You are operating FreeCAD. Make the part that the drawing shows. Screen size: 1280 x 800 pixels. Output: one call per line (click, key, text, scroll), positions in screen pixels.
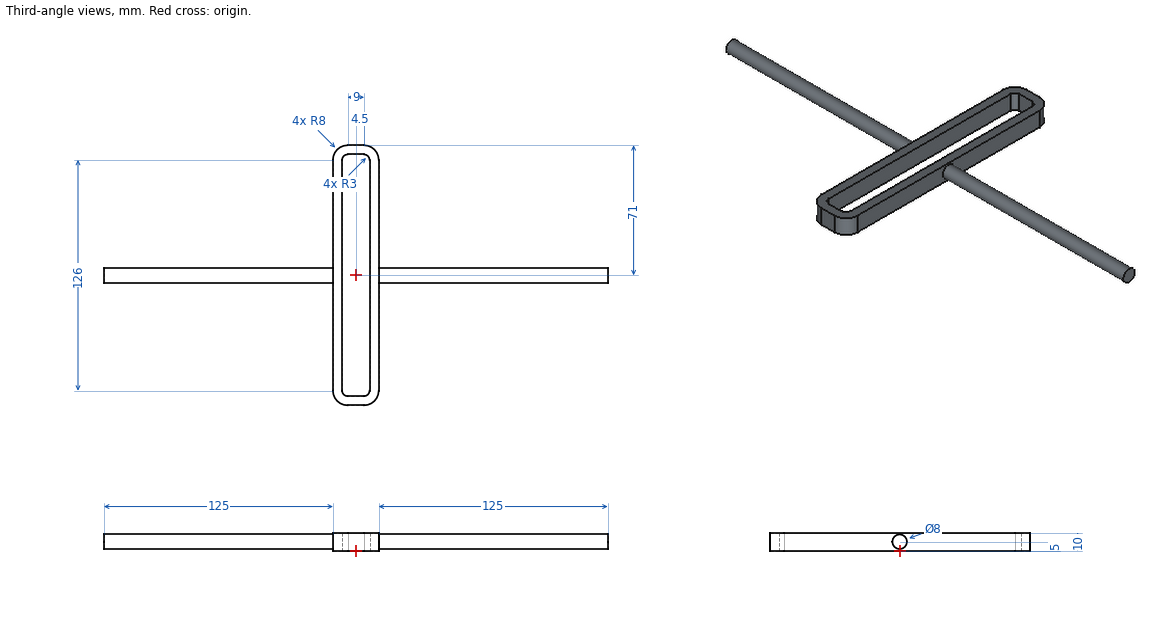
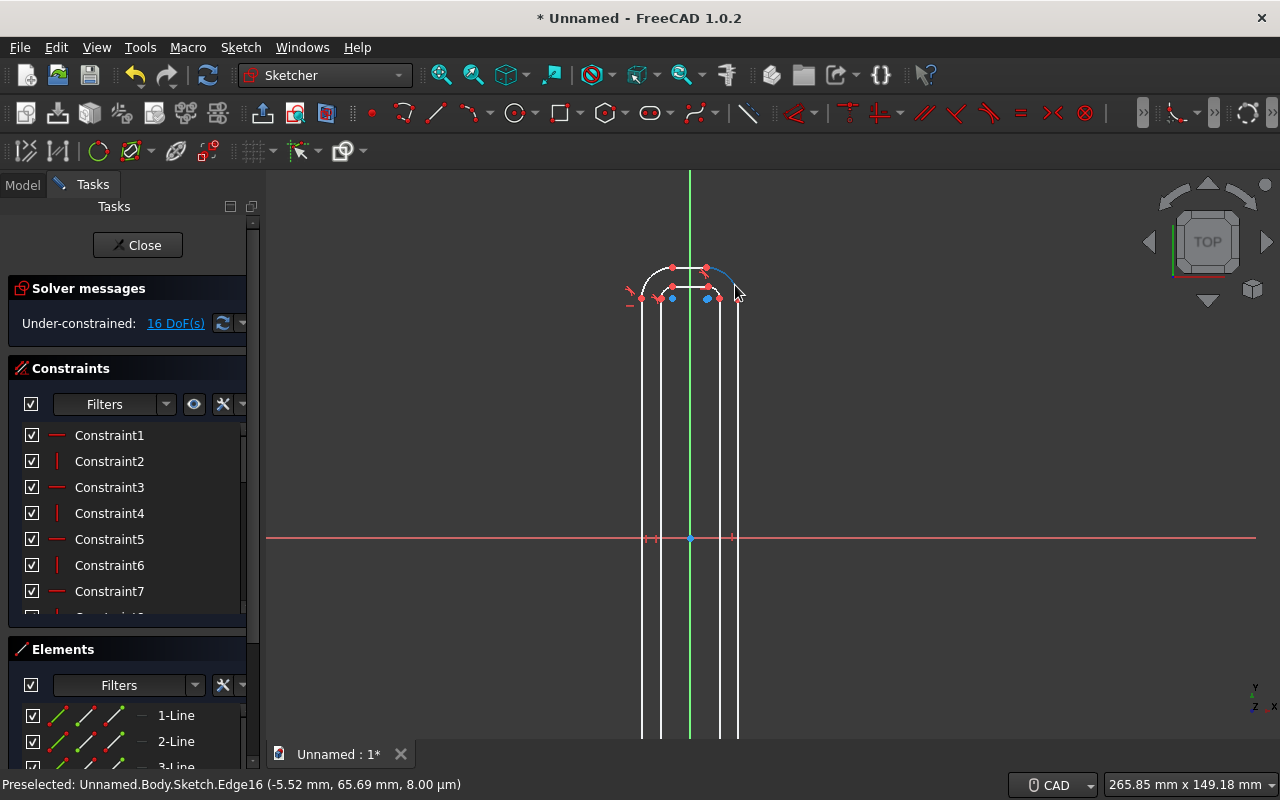
click(734, 285)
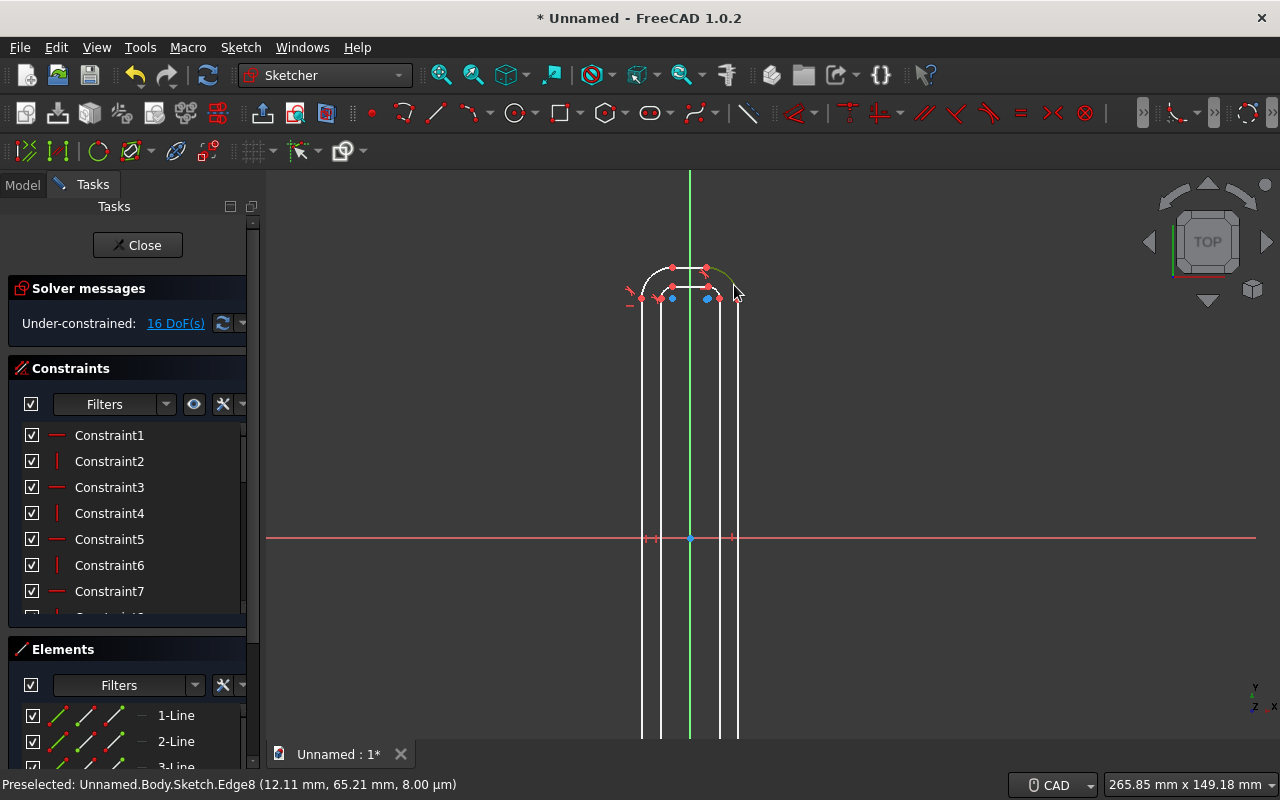
scroll(716, 290, up, 3)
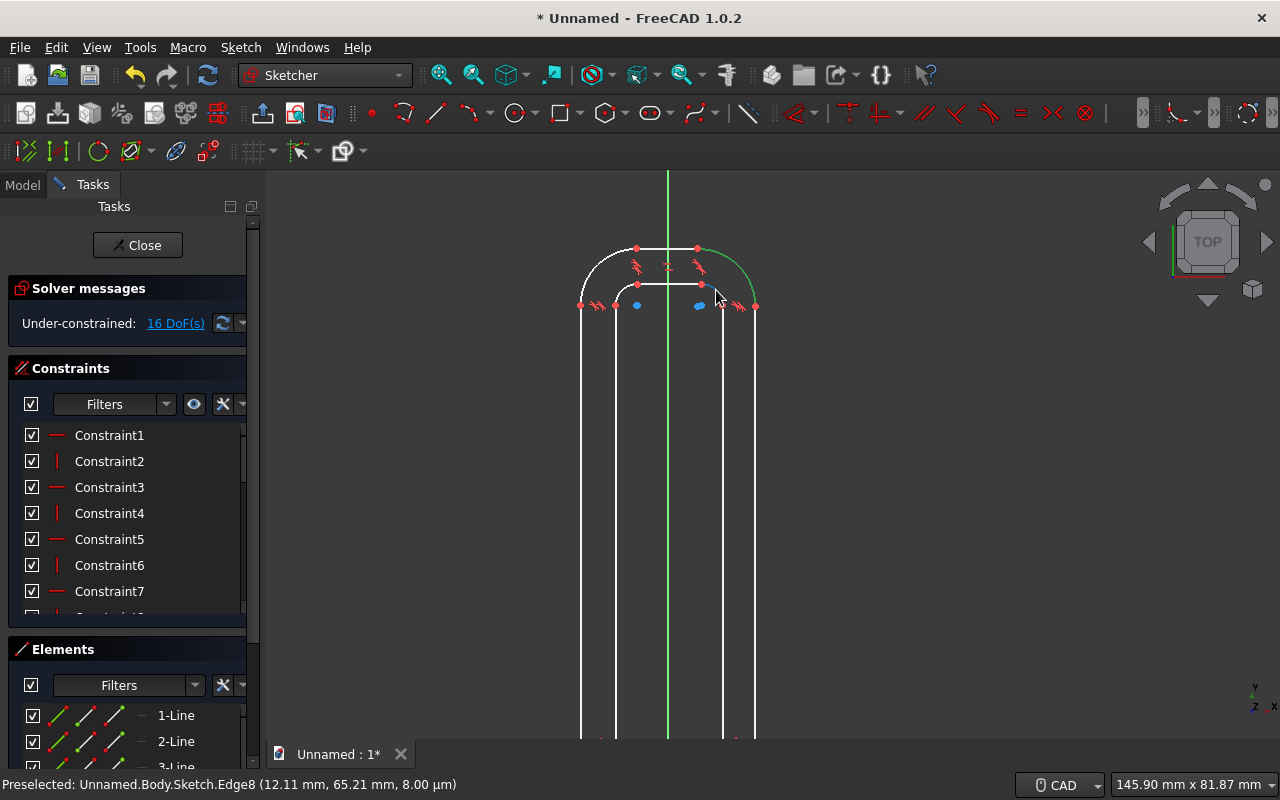
click(716, 290)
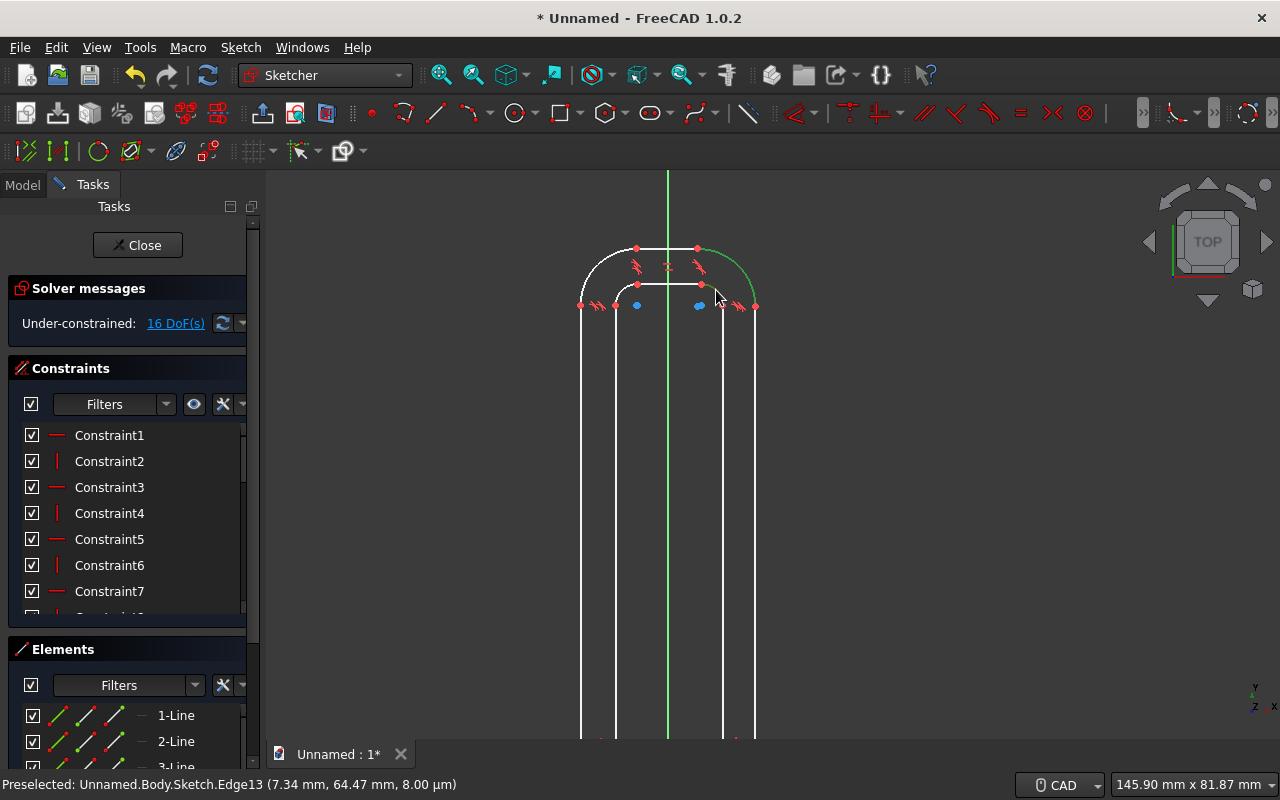
click(848, 114)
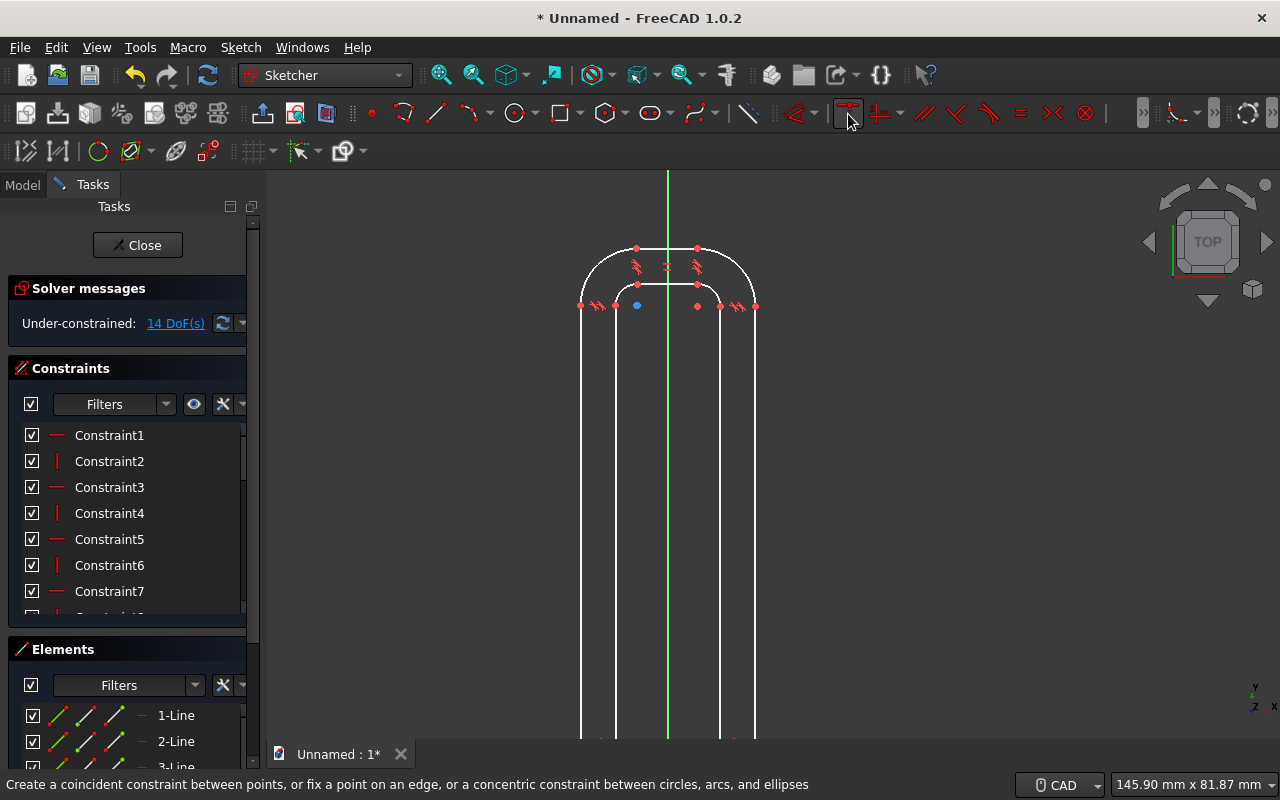
scroll(726, 287, down, 5)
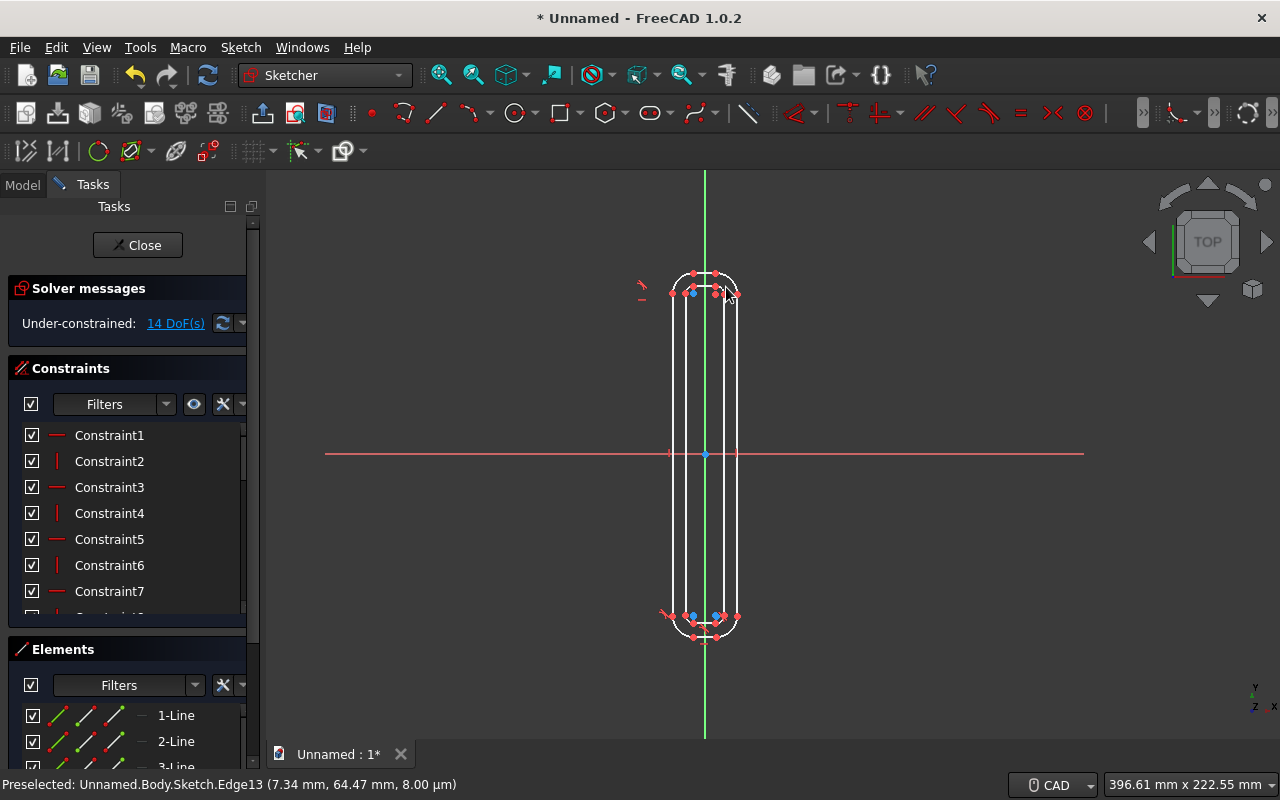
scroll(726, 635, up, 2)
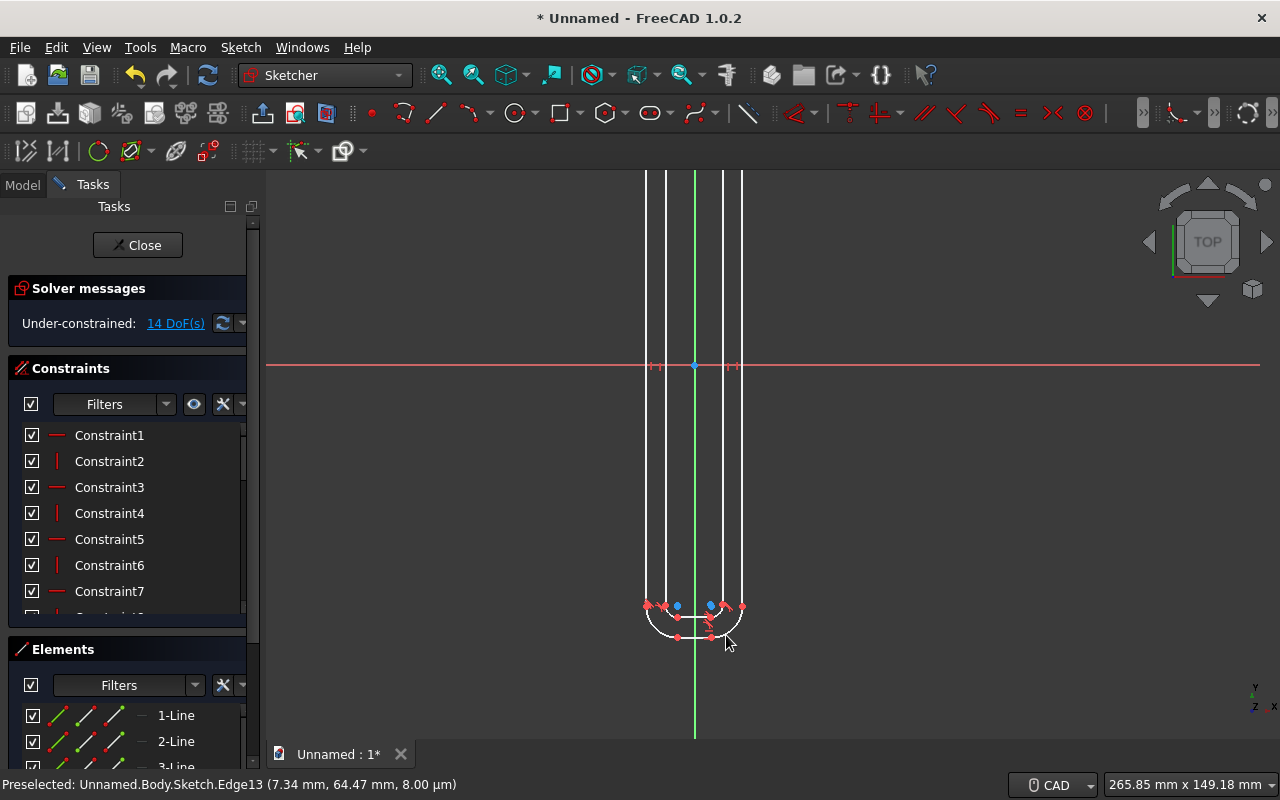
click(725, 634)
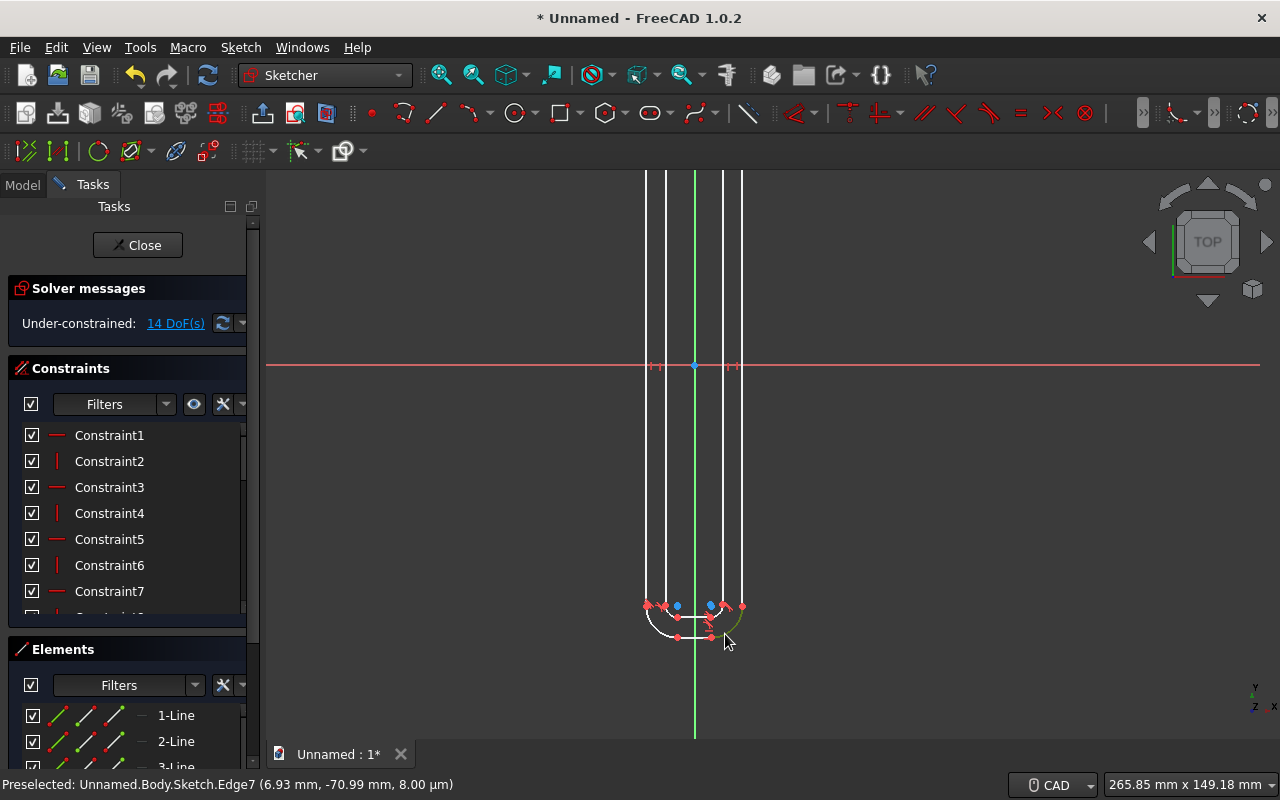
scroll(719, 614, up, 2)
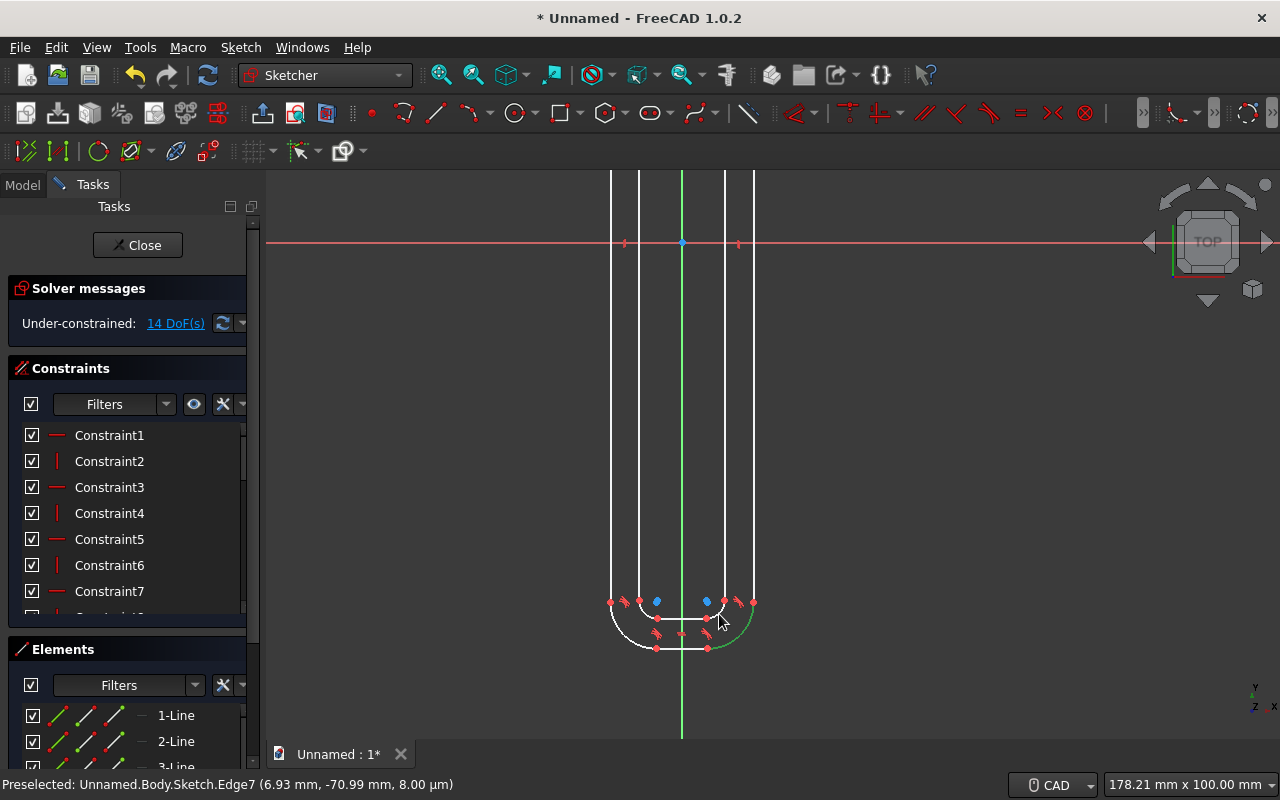
click(719, 613)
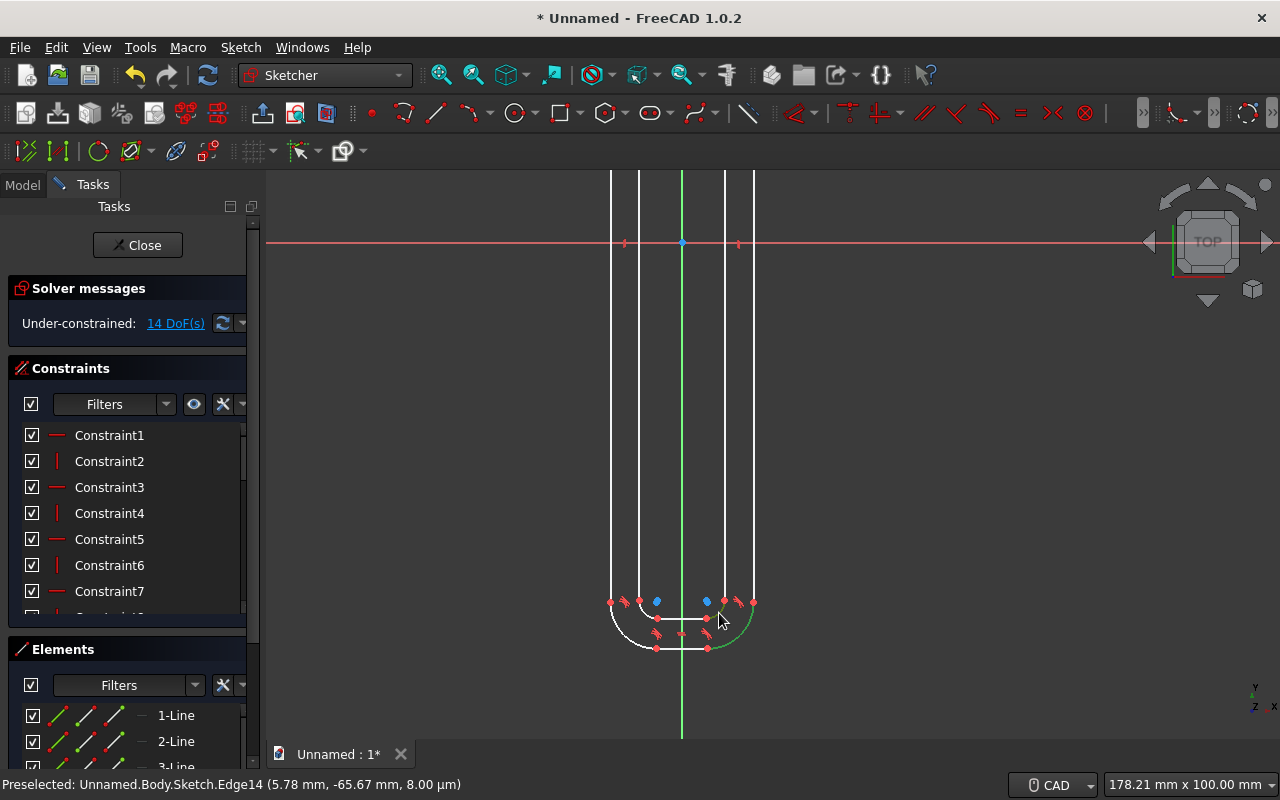
click(848, 114)